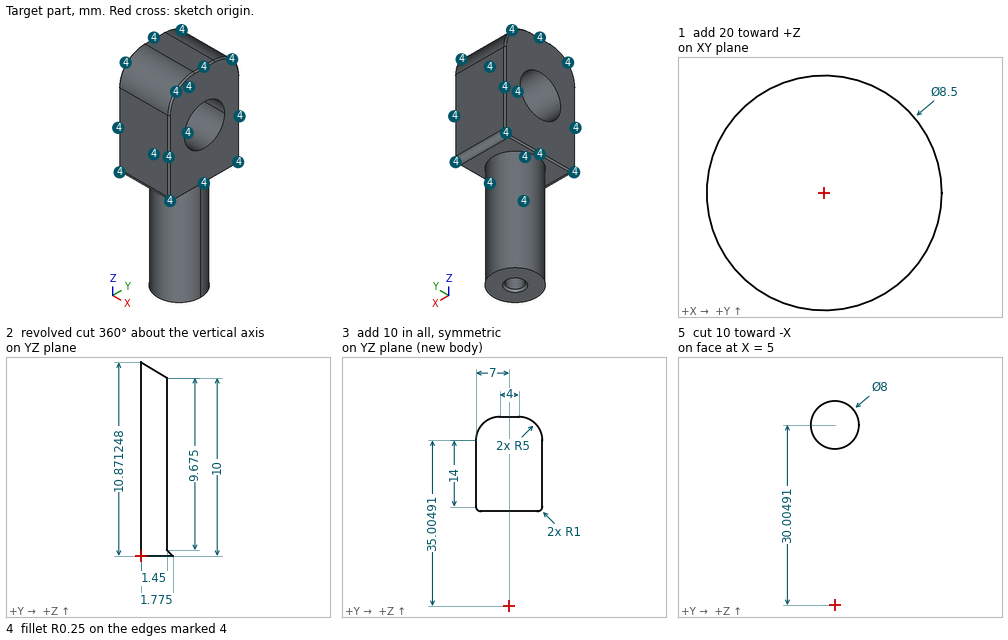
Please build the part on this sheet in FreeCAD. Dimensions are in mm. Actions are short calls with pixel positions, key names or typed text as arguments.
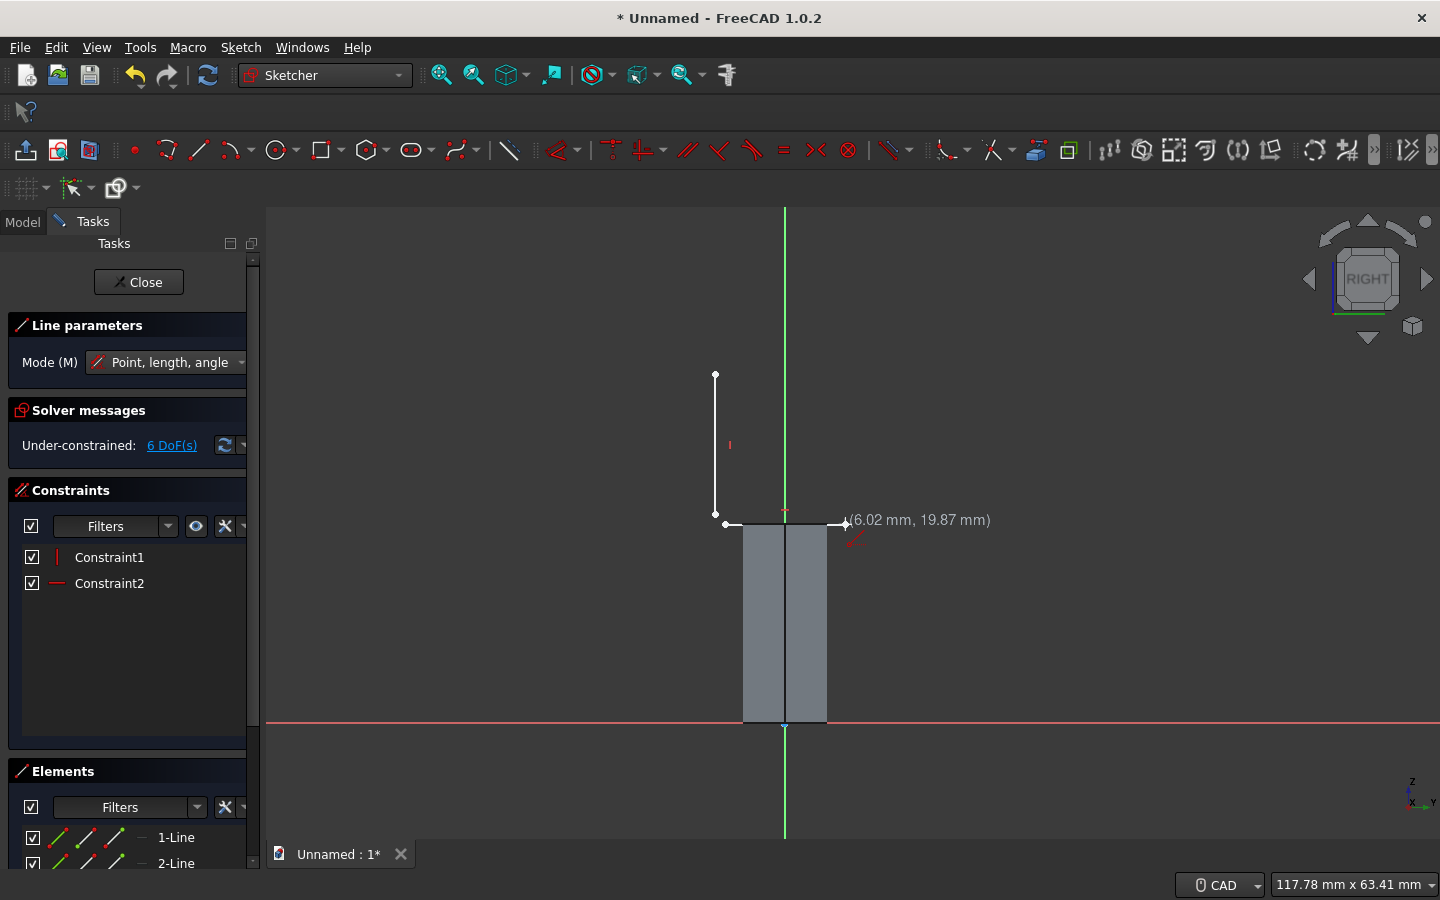
click(855, 514)
click(855, 374)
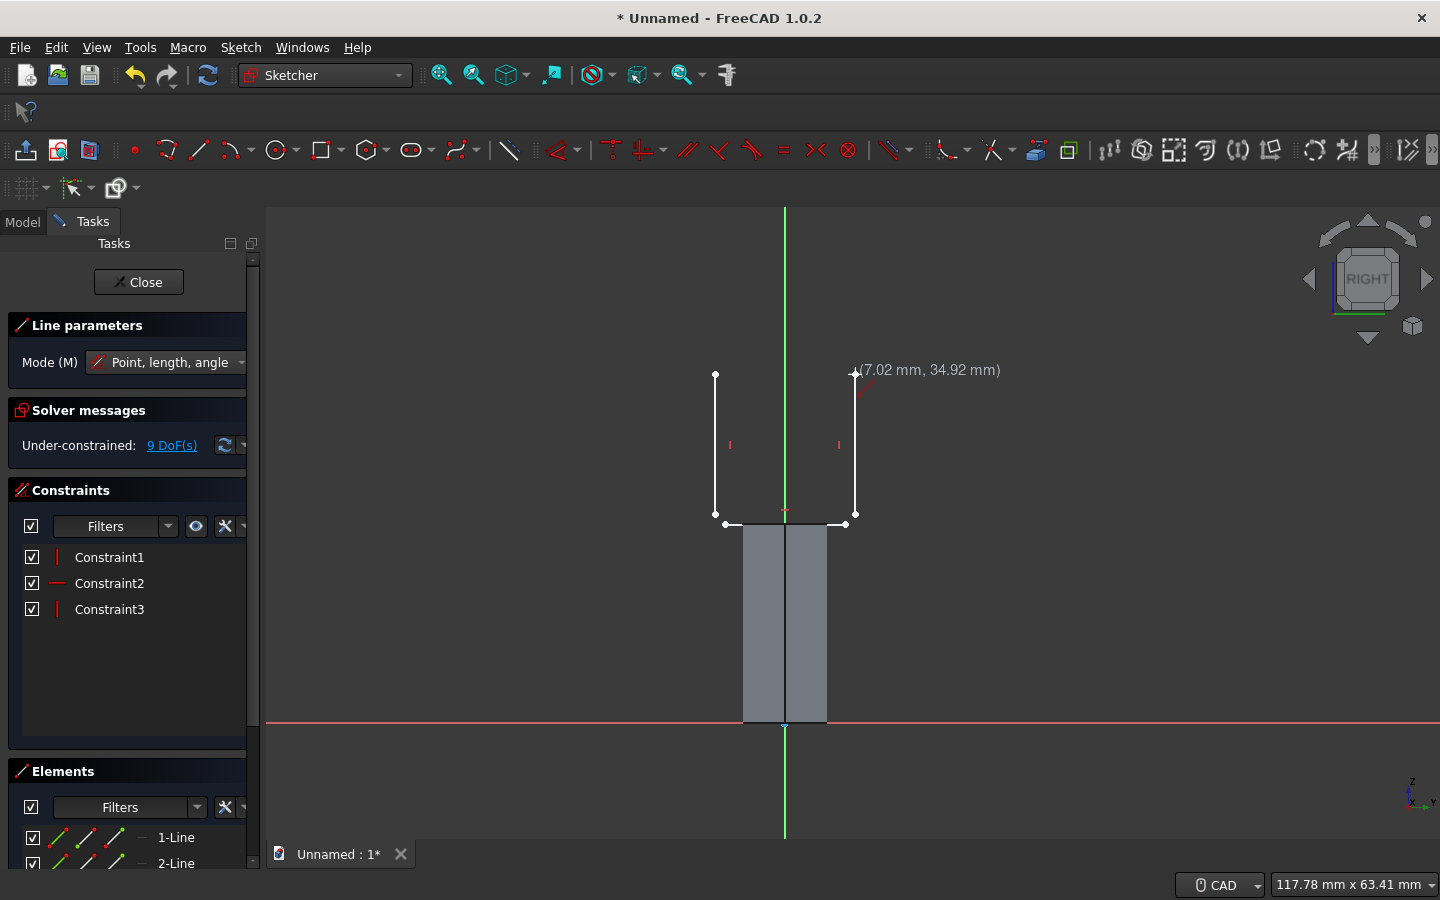
click(805, 324)
click(765, 324)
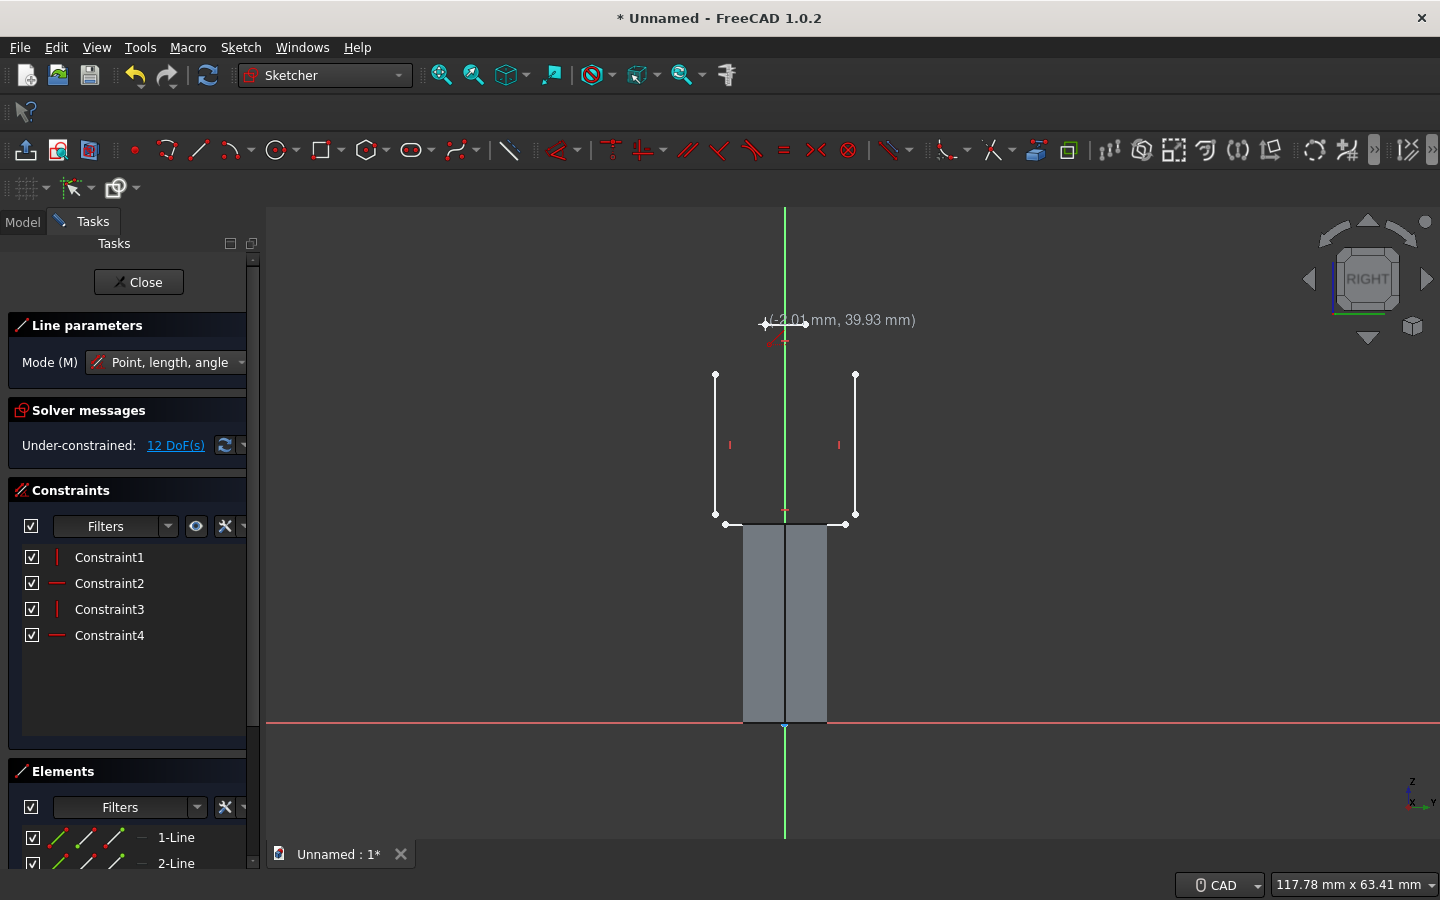
key(g)
key(3)
key(a)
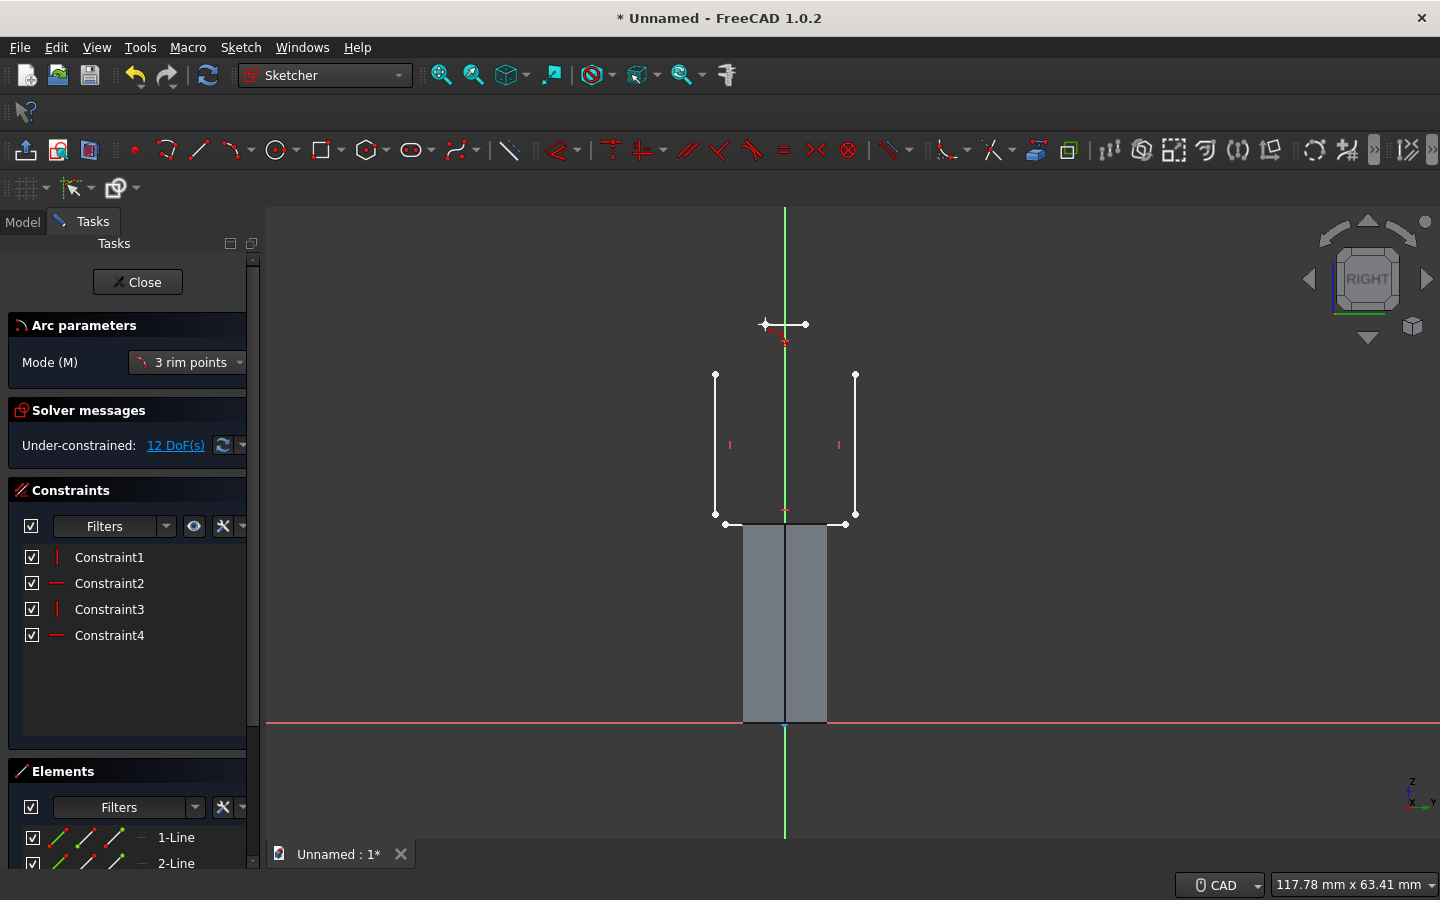
click(715, 515)
click(725, 525)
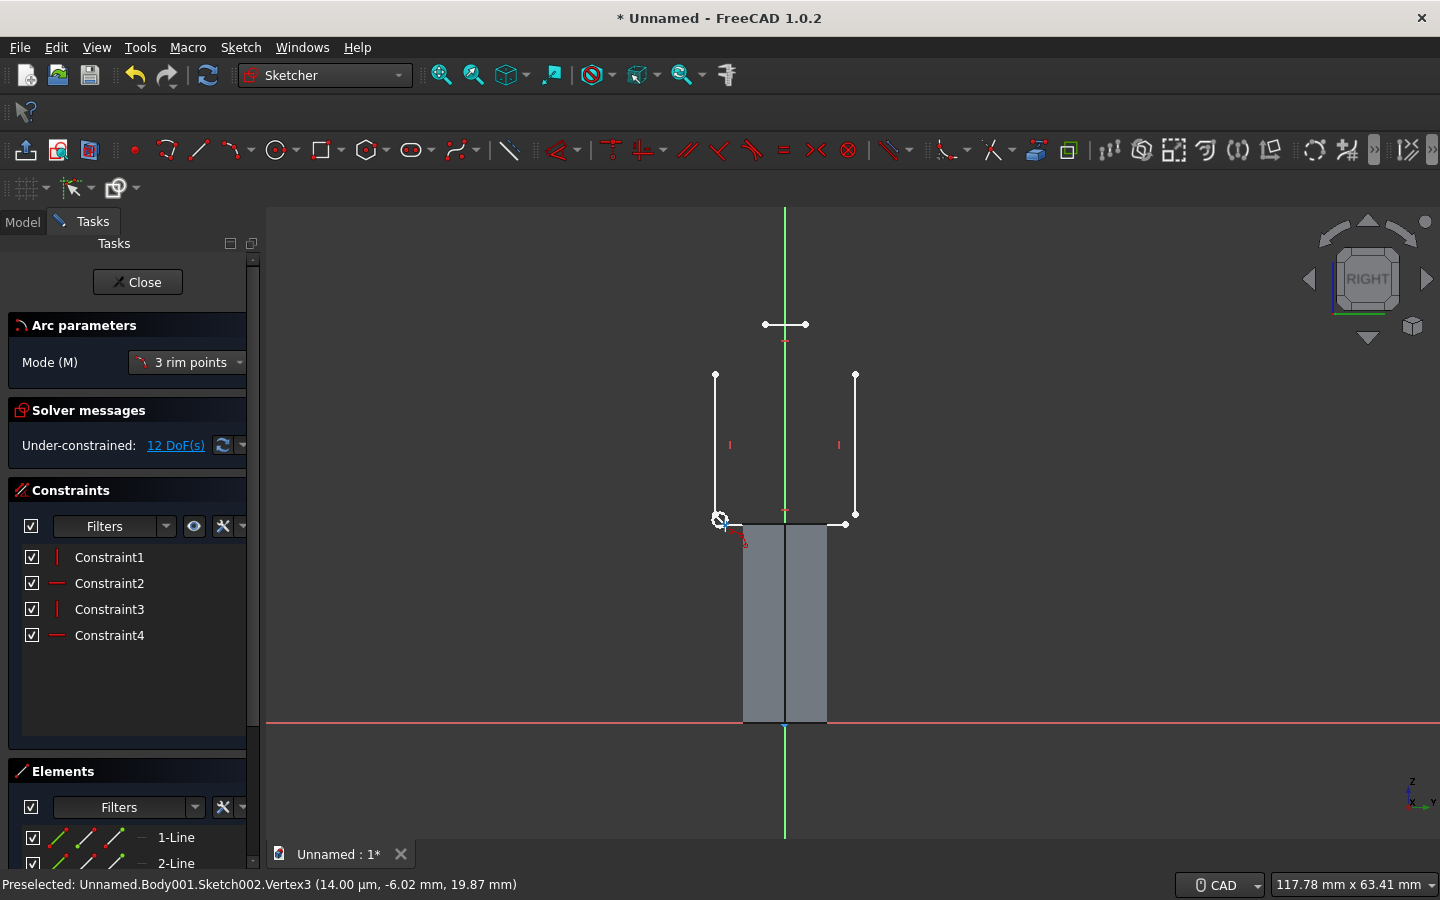
scroll(718, 521, up, 9)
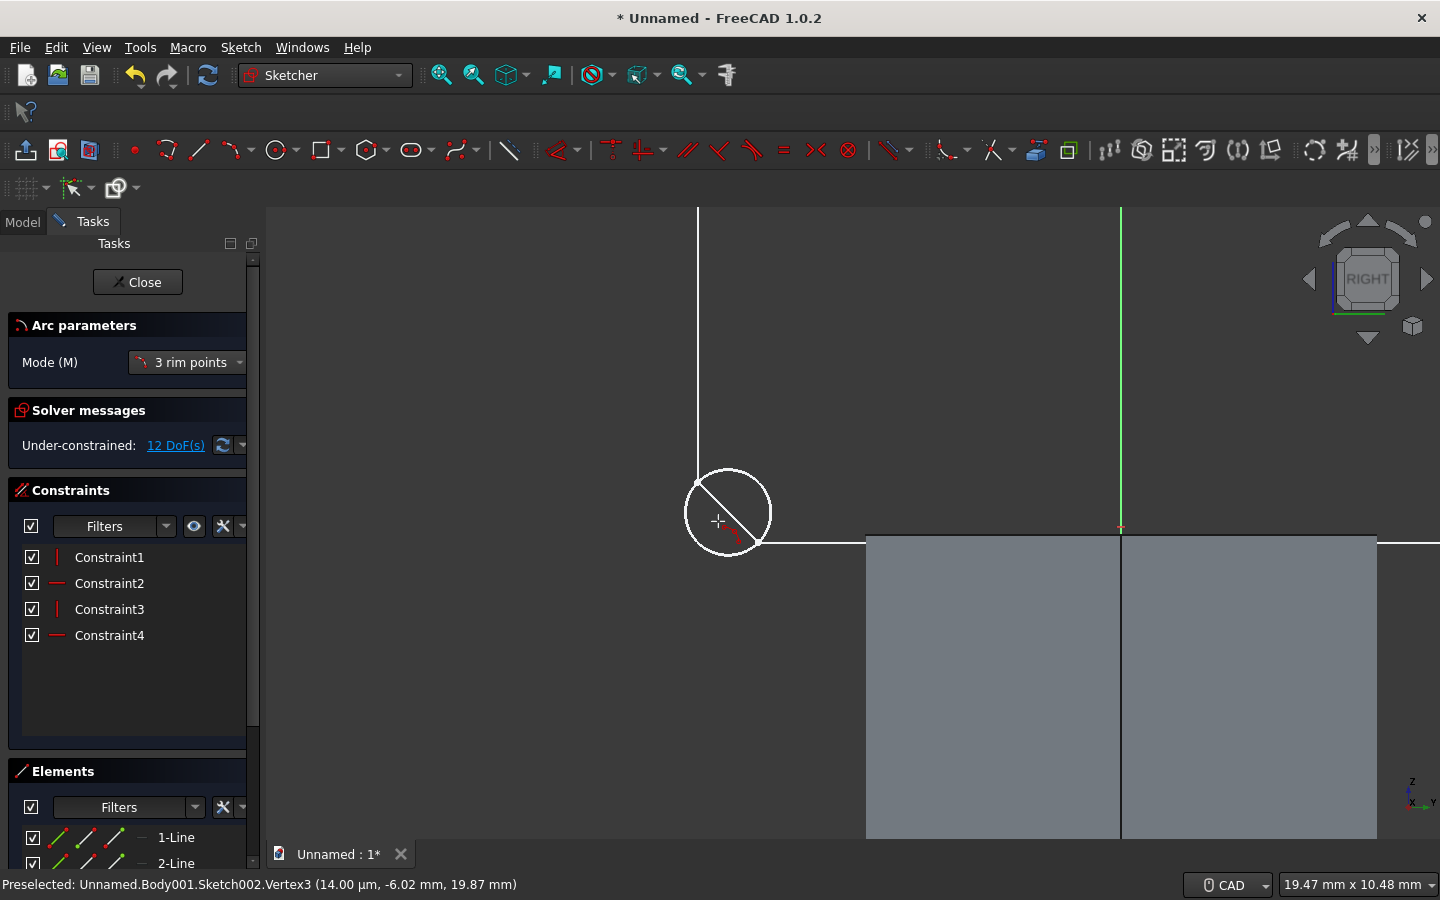
click(717, 517)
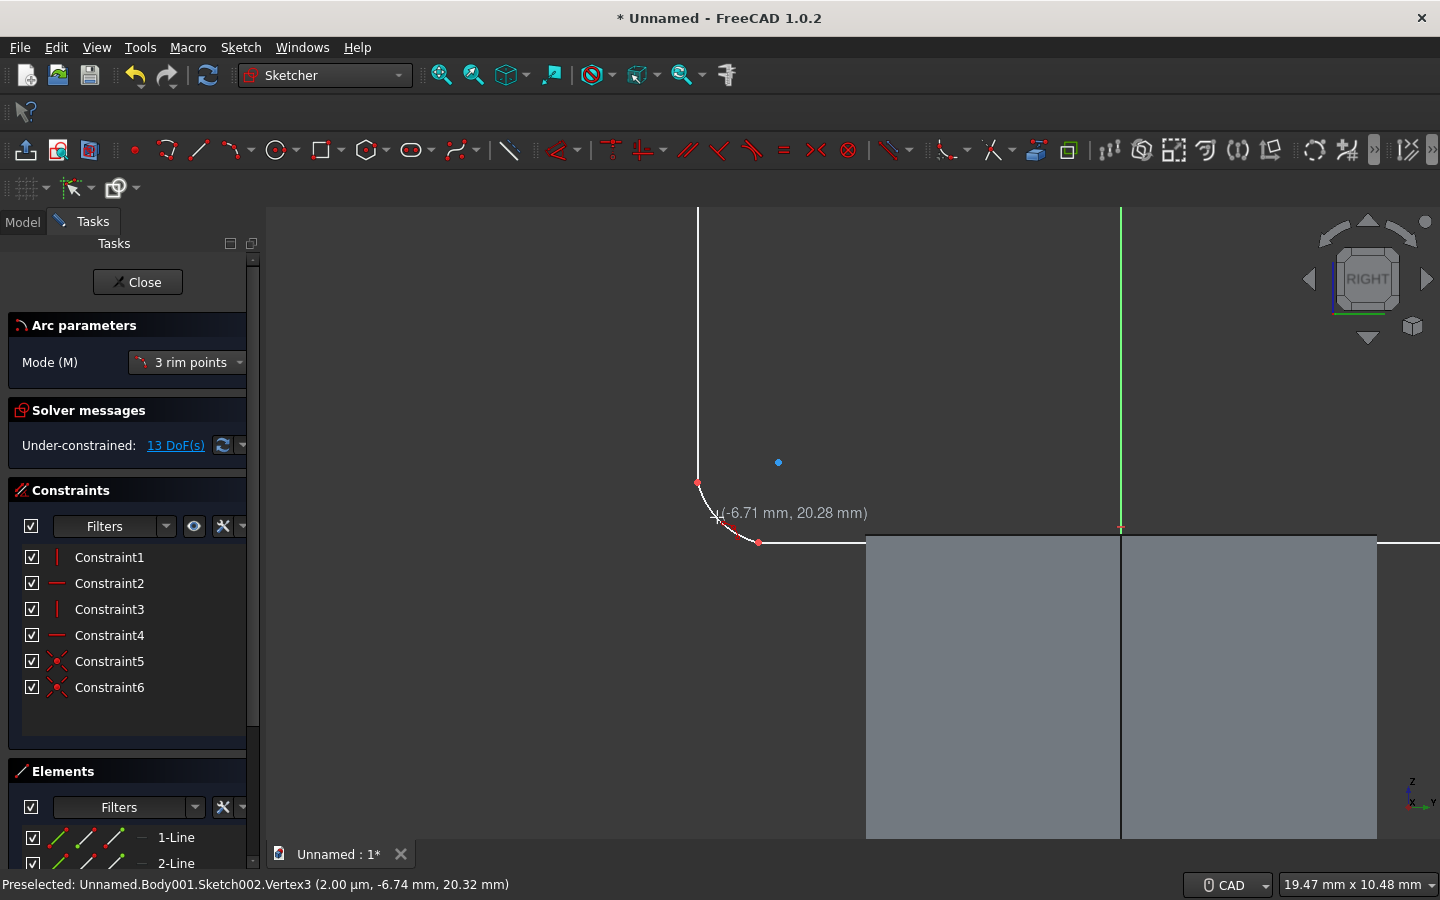
scroll(718, 521, down, 9)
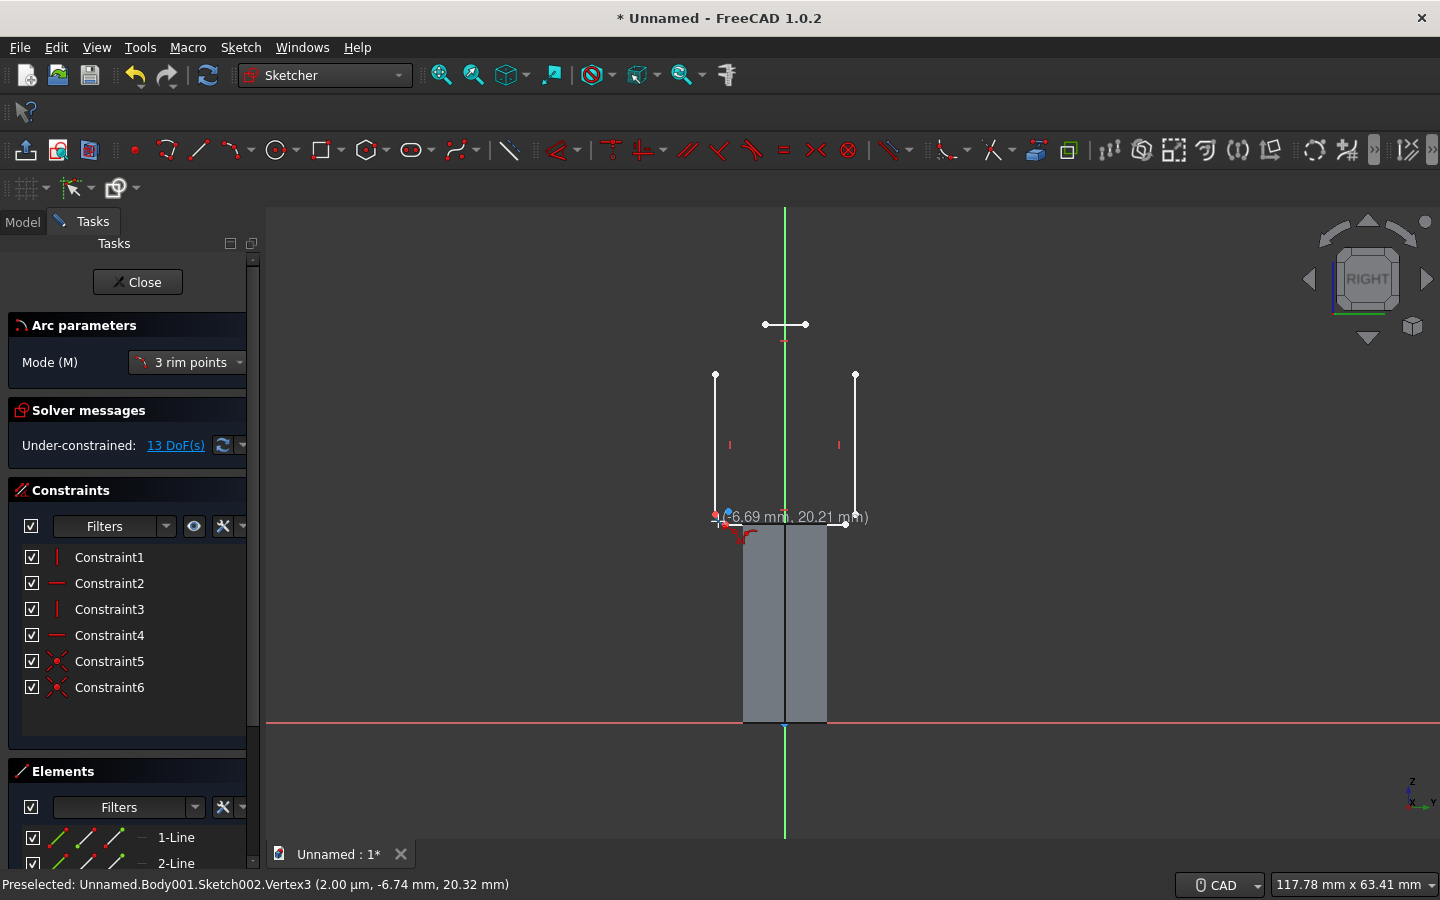
click(845, 525)
click(855, 515)